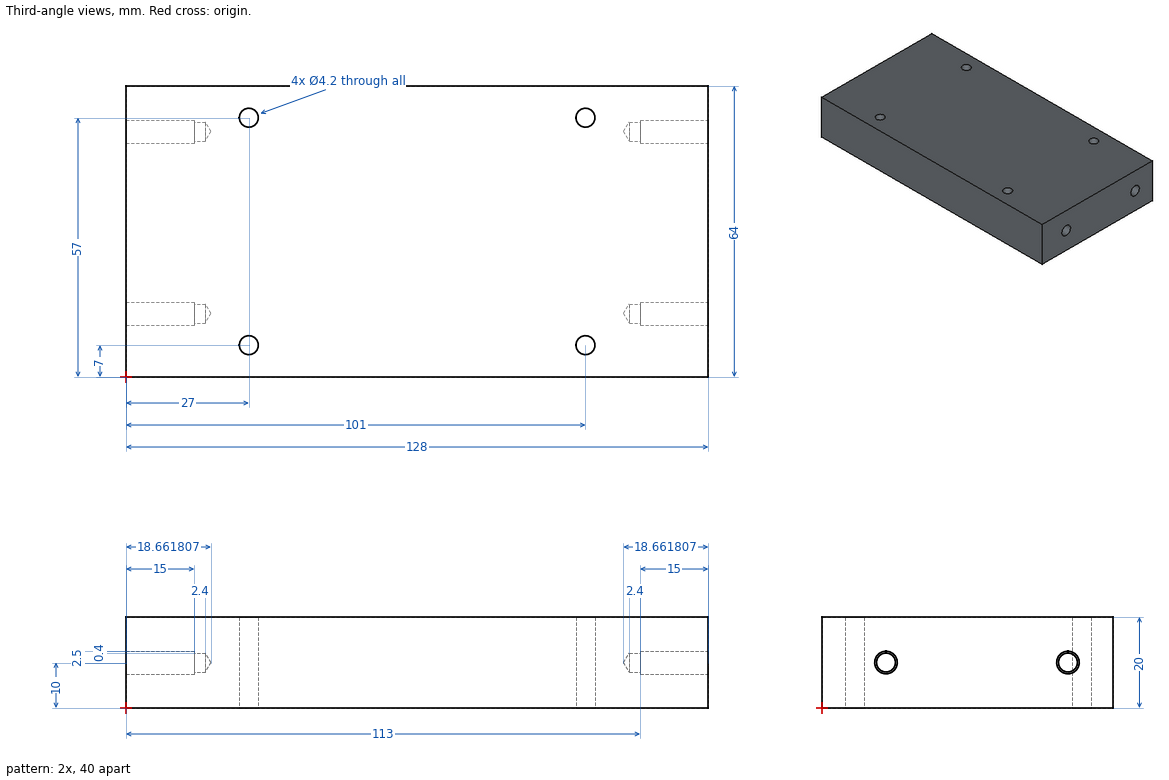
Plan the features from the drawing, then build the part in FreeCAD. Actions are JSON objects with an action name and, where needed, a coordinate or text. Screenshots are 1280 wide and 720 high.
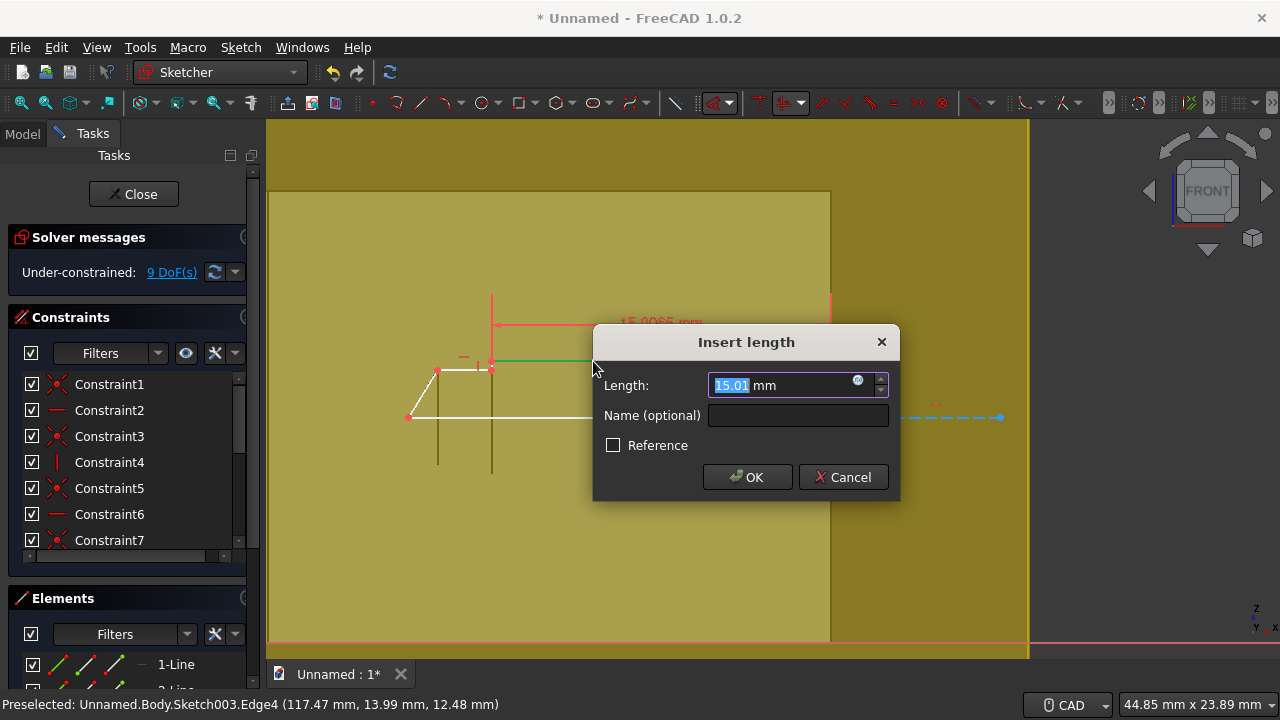
{"action": "type", "text": "15"}
{"action": "key", "text": "Return"}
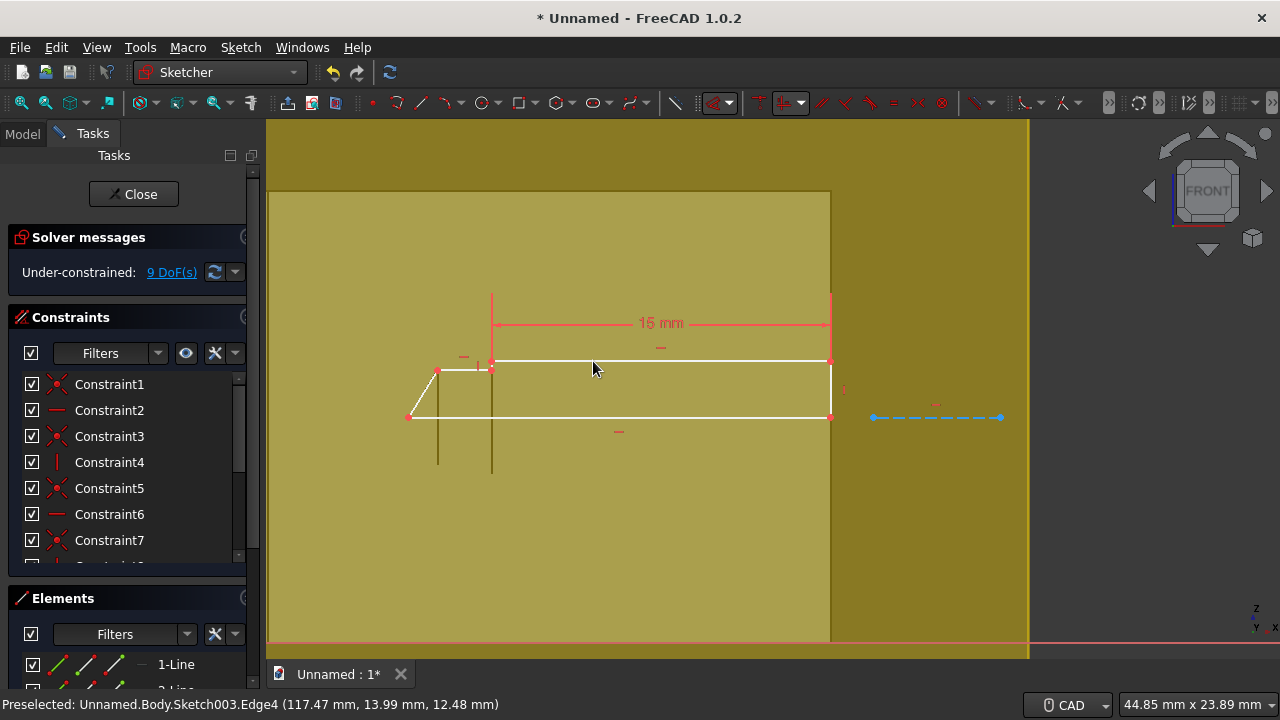
{"action": "left_click", "coordinate": [454, 370]}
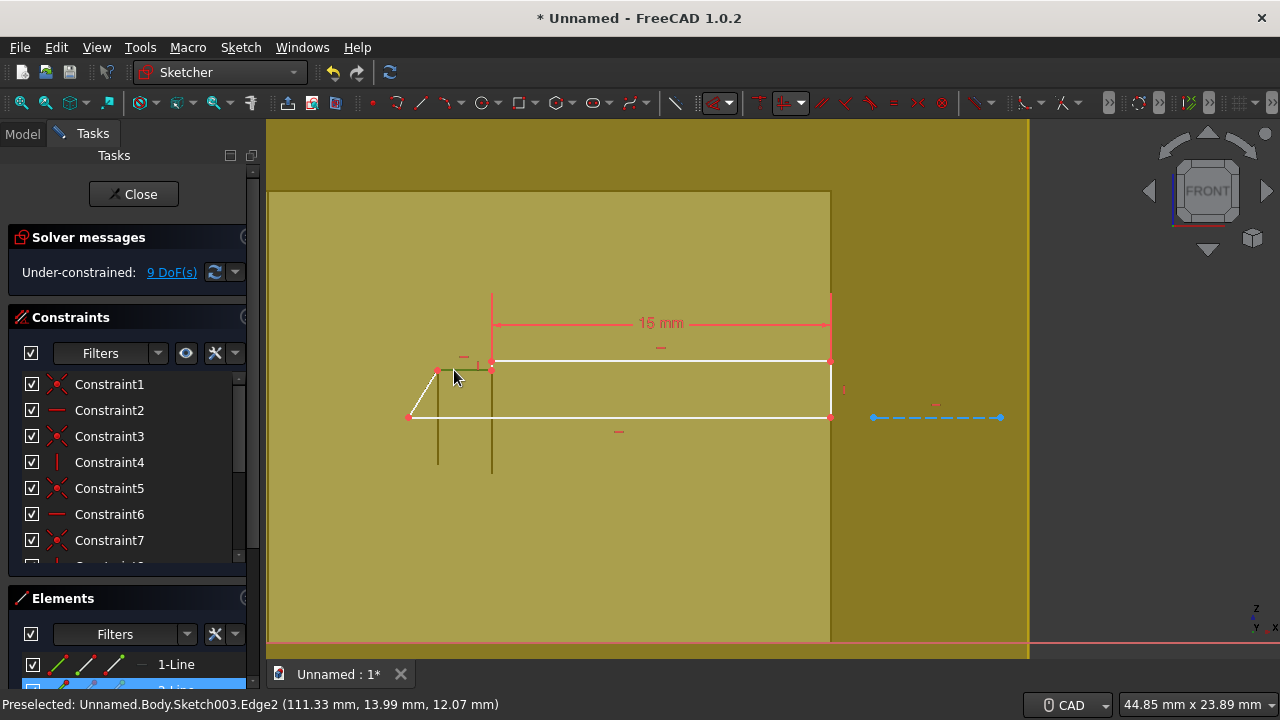
{"action": "key", "text": "l"}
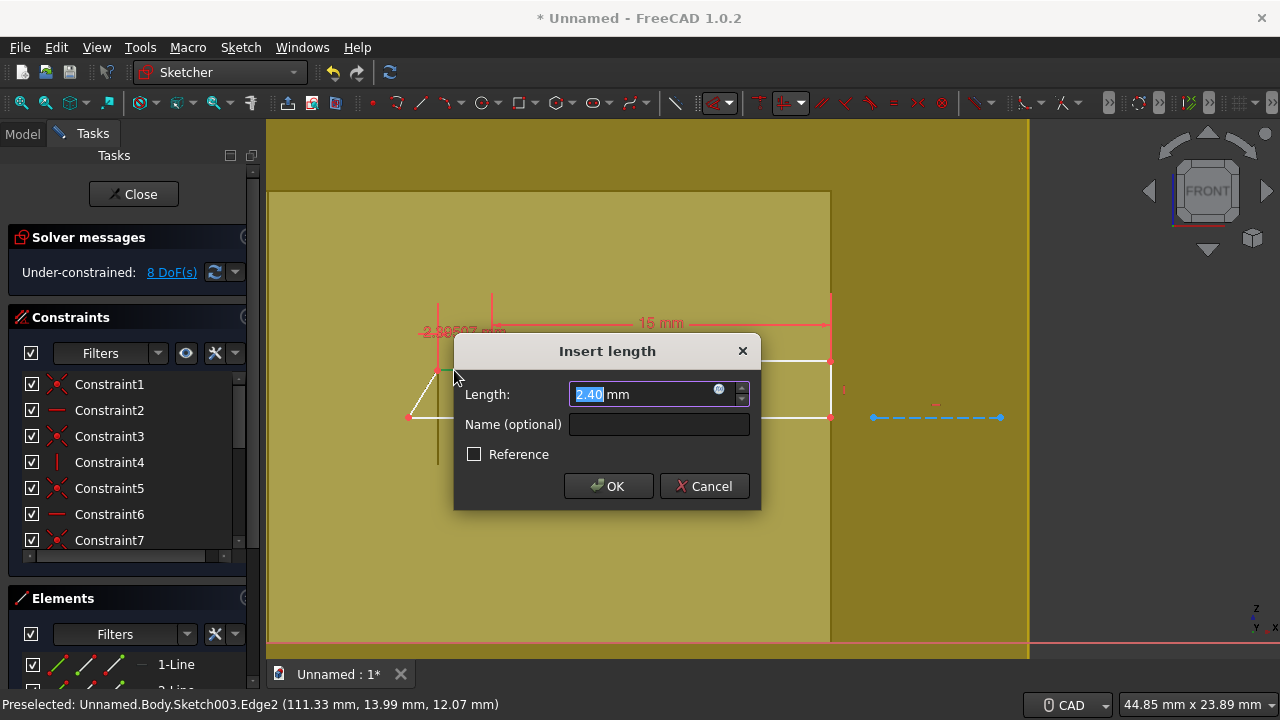
{"action": "type", "text": "2.4"}
{"action": "key", "text": "Return"}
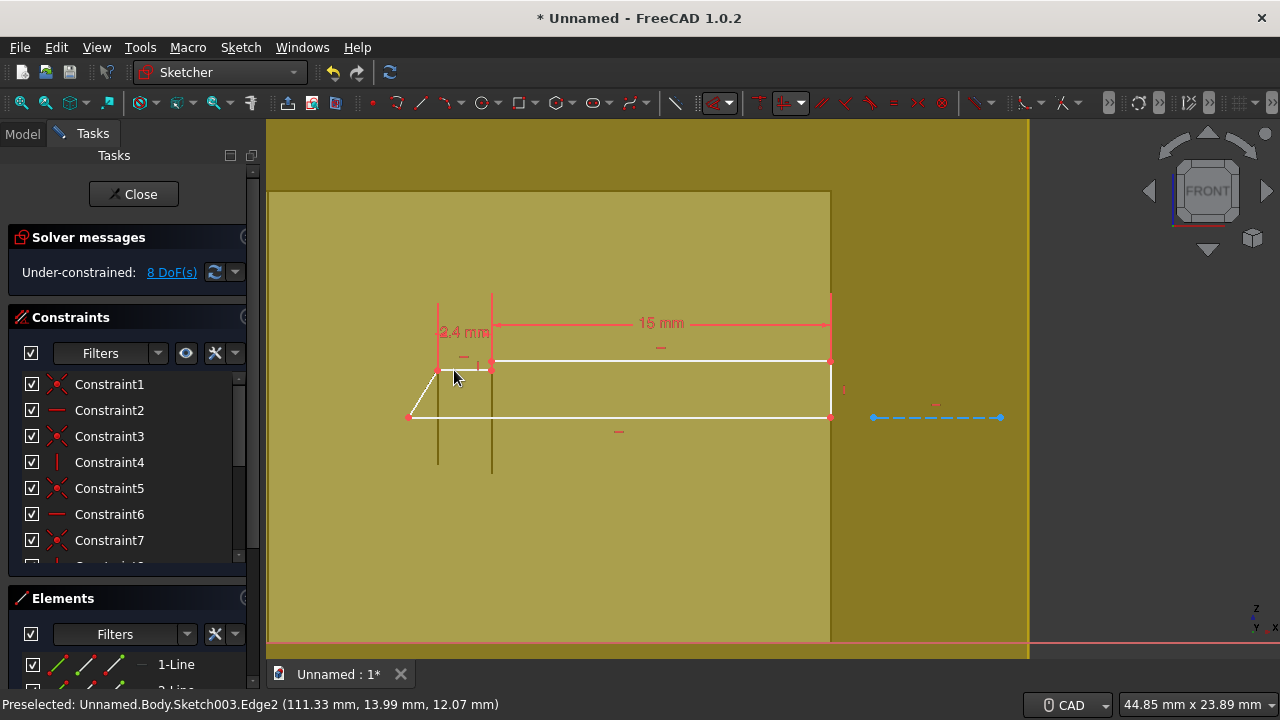
{"action": "scroll", "coordinate": [492, 366], "scroll_direction": "up", "scroll_amount": 8}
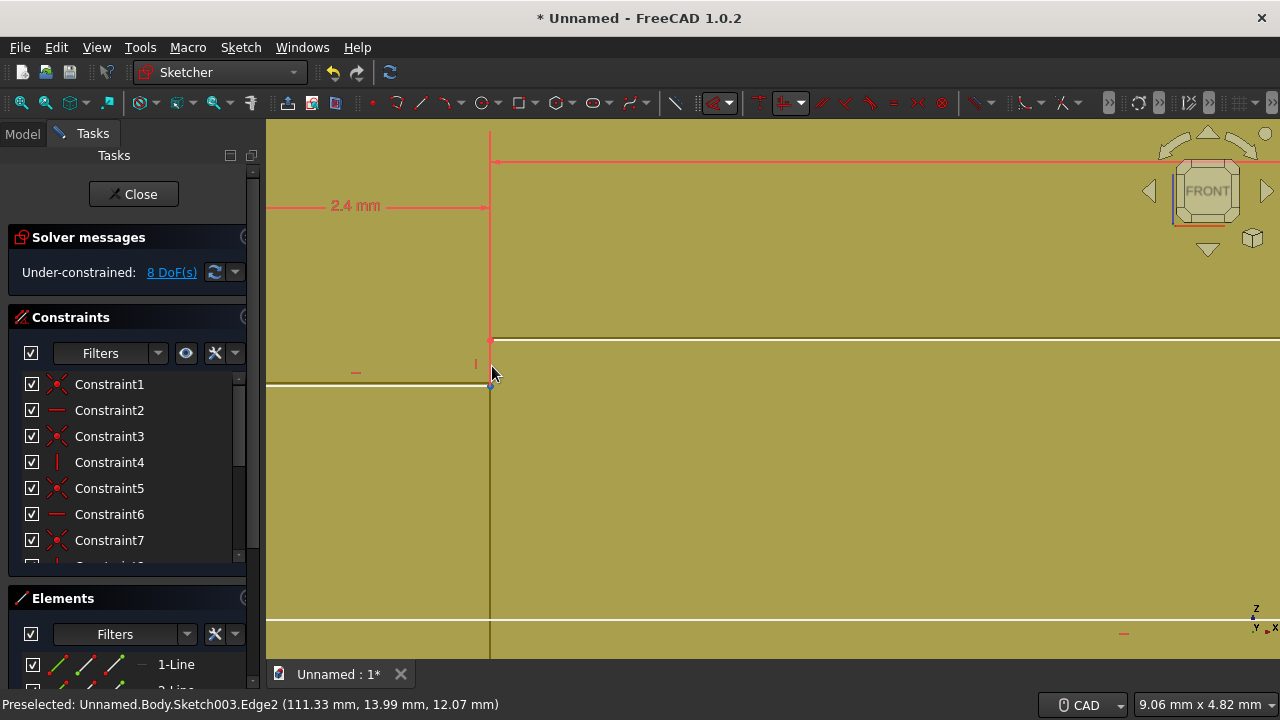
{"action": "left_click", "coordinate": [490, 363]}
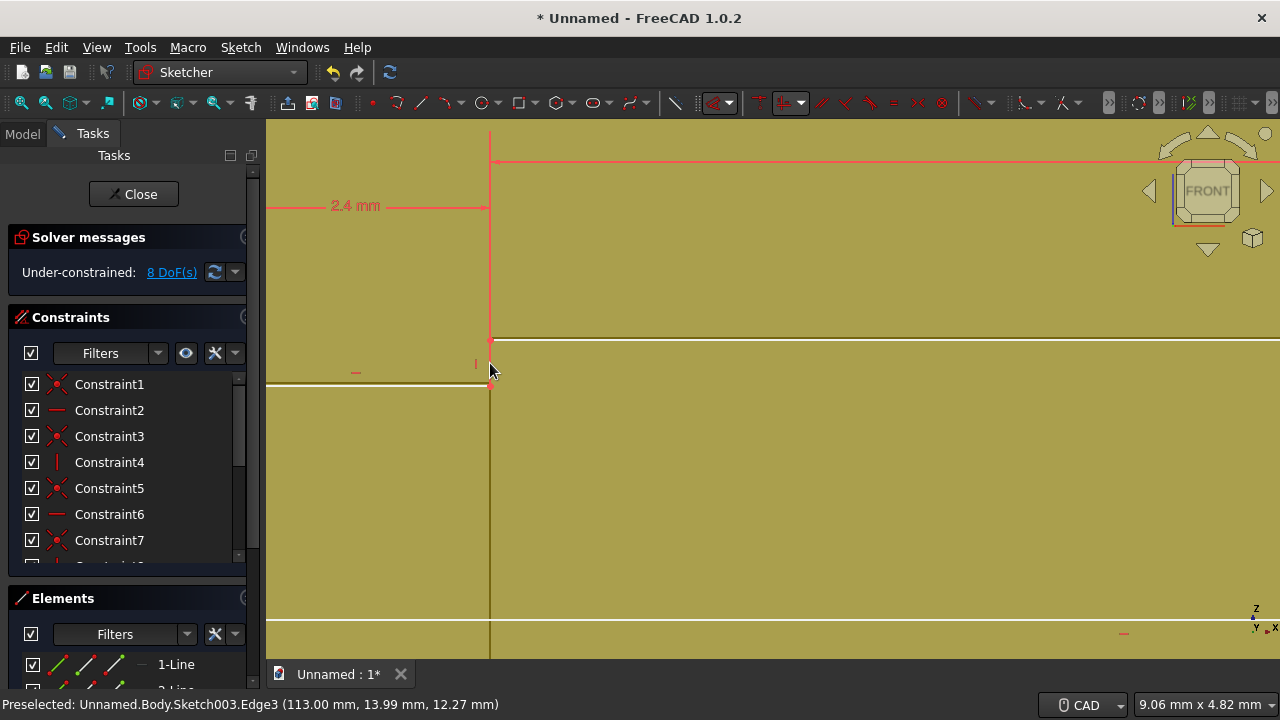
{"action": "key", "text": "i"}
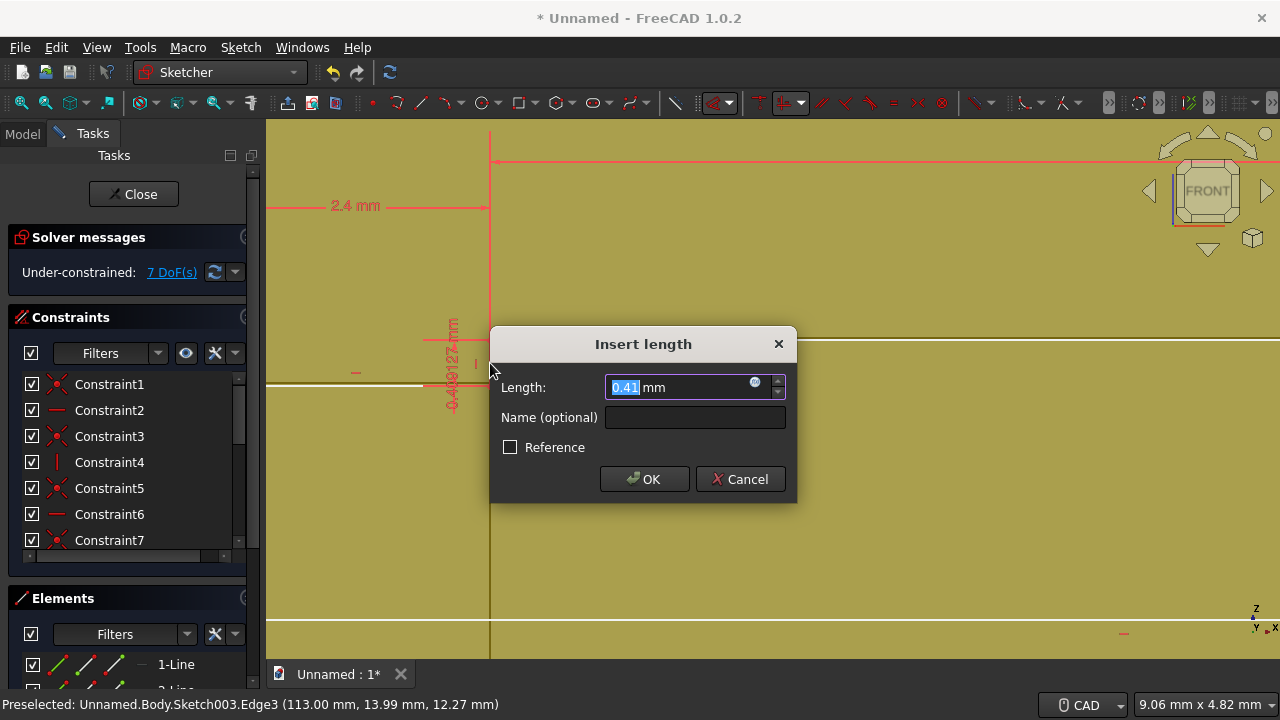
{"action": "type", "text": "0.4"}
{"action": "key", "text": "Return"}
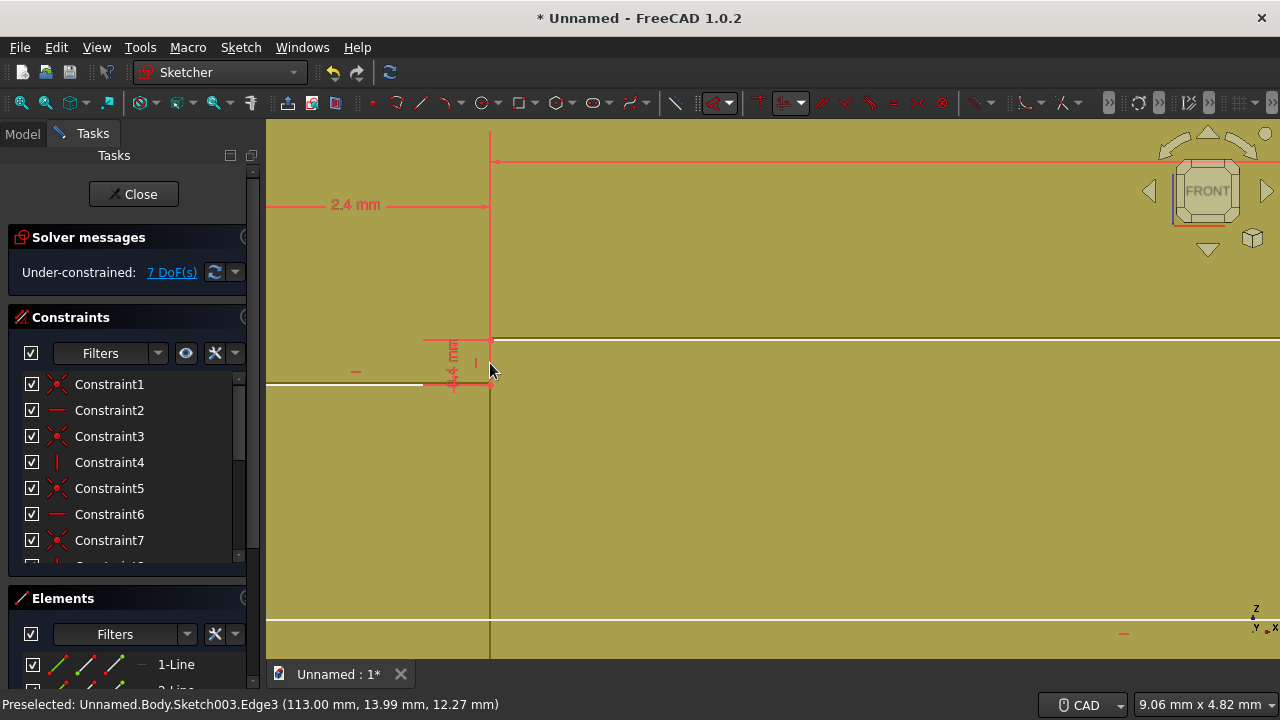
{"action": "scroll", "coordinate": [492, 366], "scroll_direction": "down", "scroll_amount": 8}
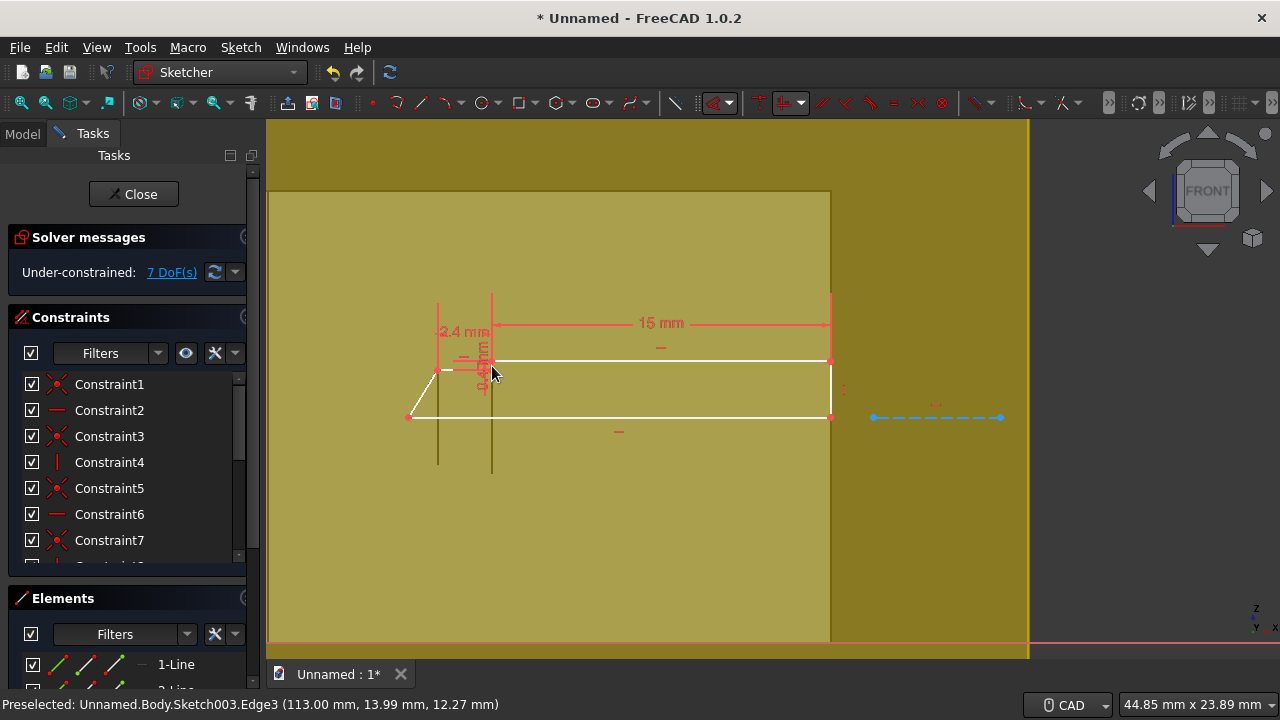
{"action": "left_click", "coordinate": [831, 378]}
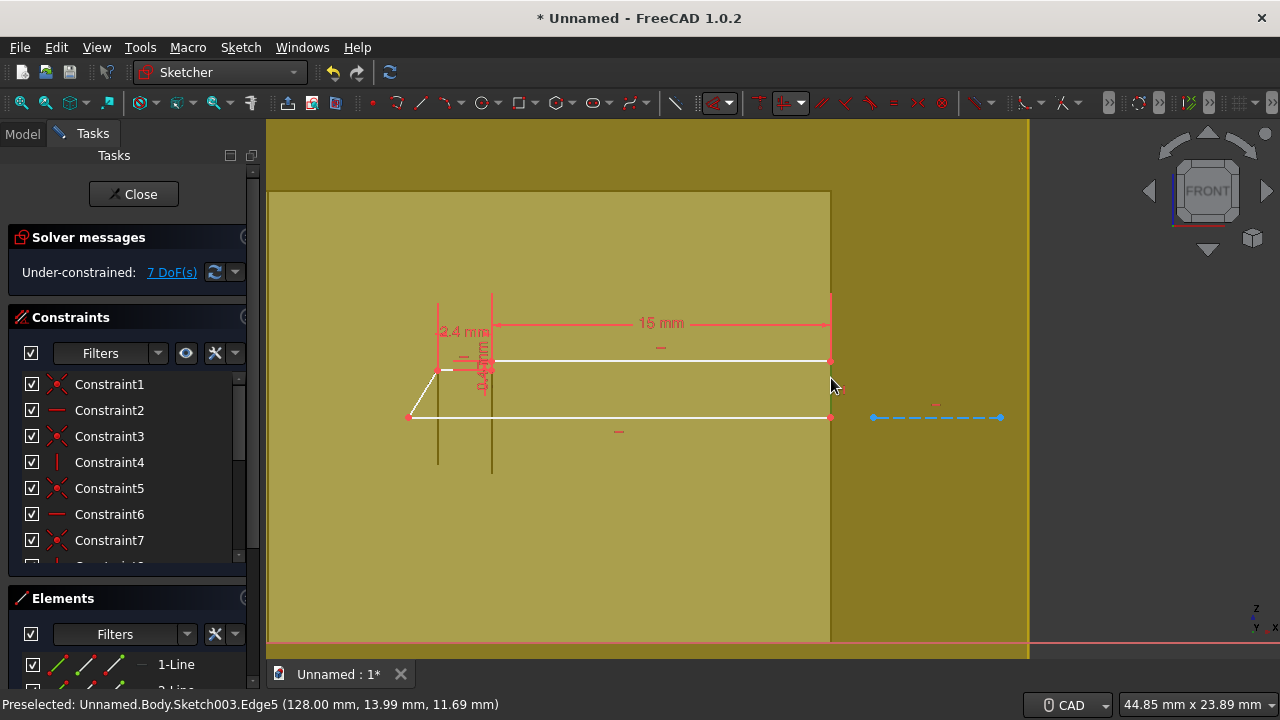
{"action": "key", "text": "i"}